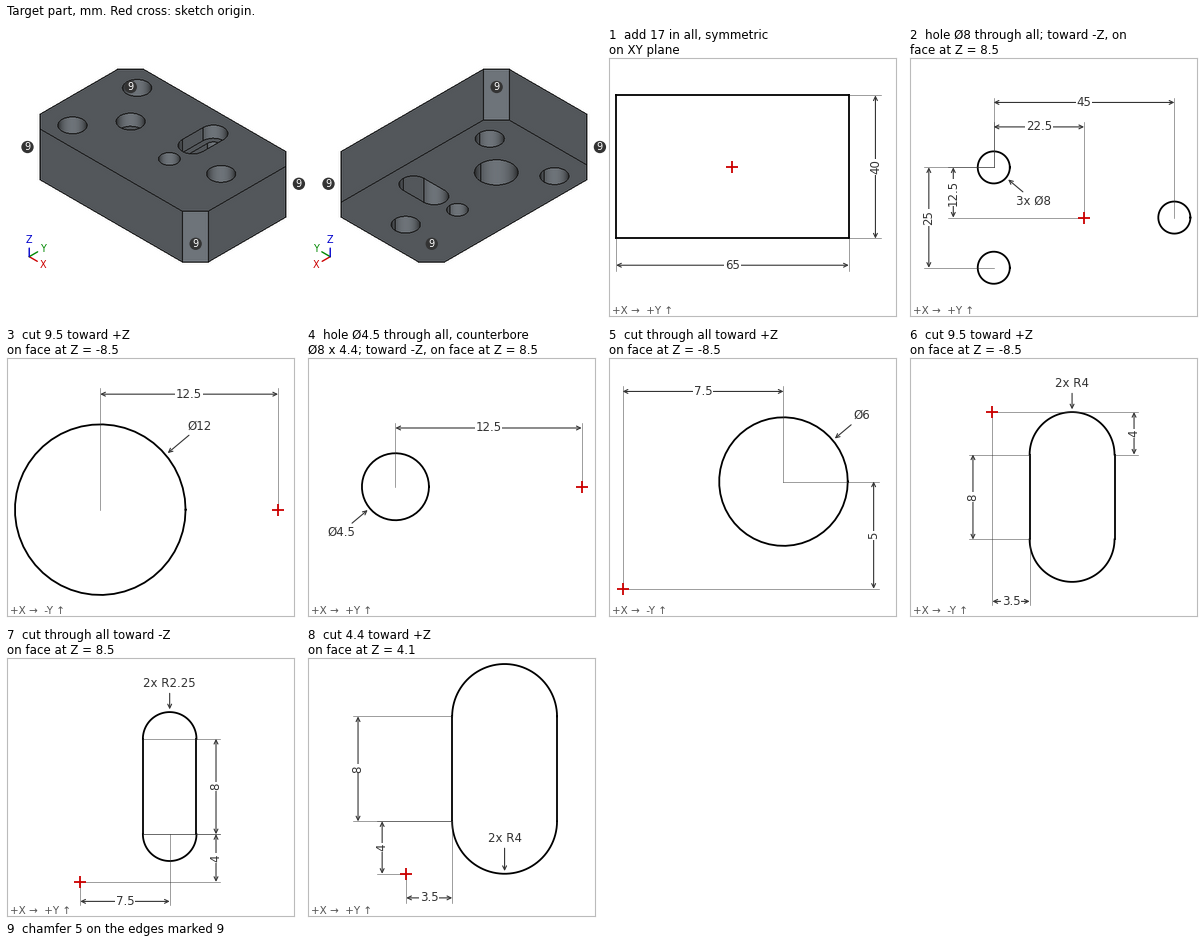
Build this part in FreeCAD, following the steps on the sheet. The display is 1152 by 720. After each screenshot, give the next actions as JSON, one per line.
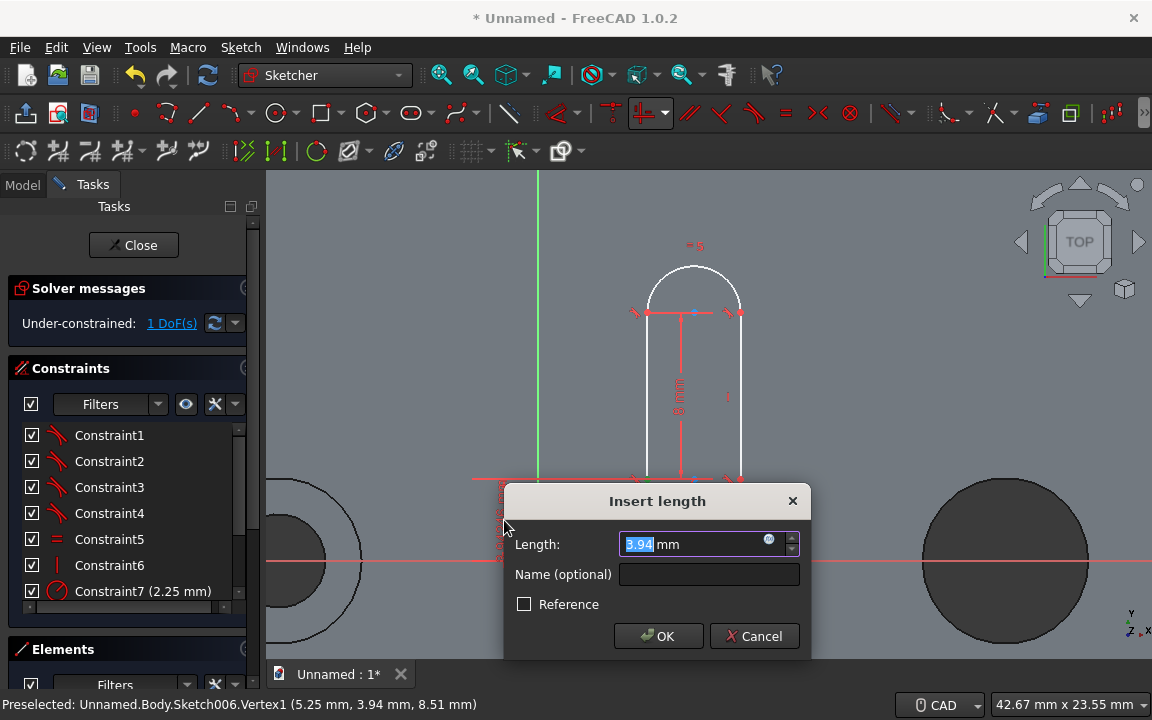
{"action": "type", "text": "4"}
{"action": "key", "text": "Return"}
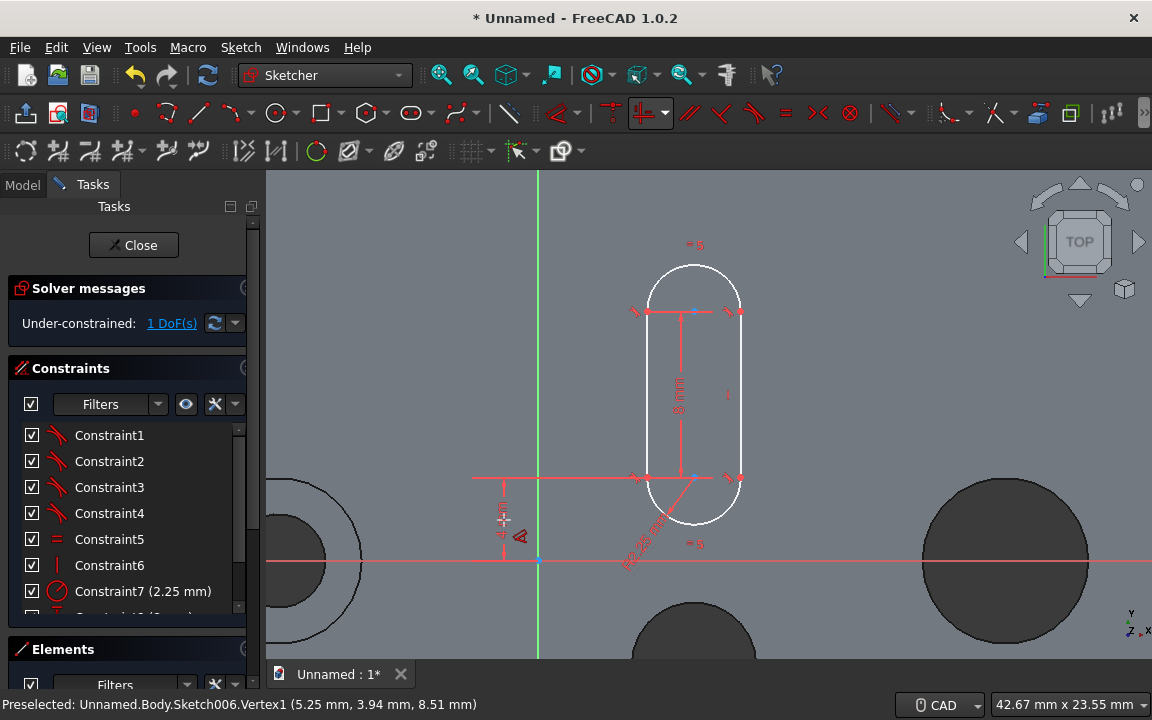
{"action": "left_click", "coordinate": [694, 478]}
{"action": "left_click", "coordinate": [616, 595]}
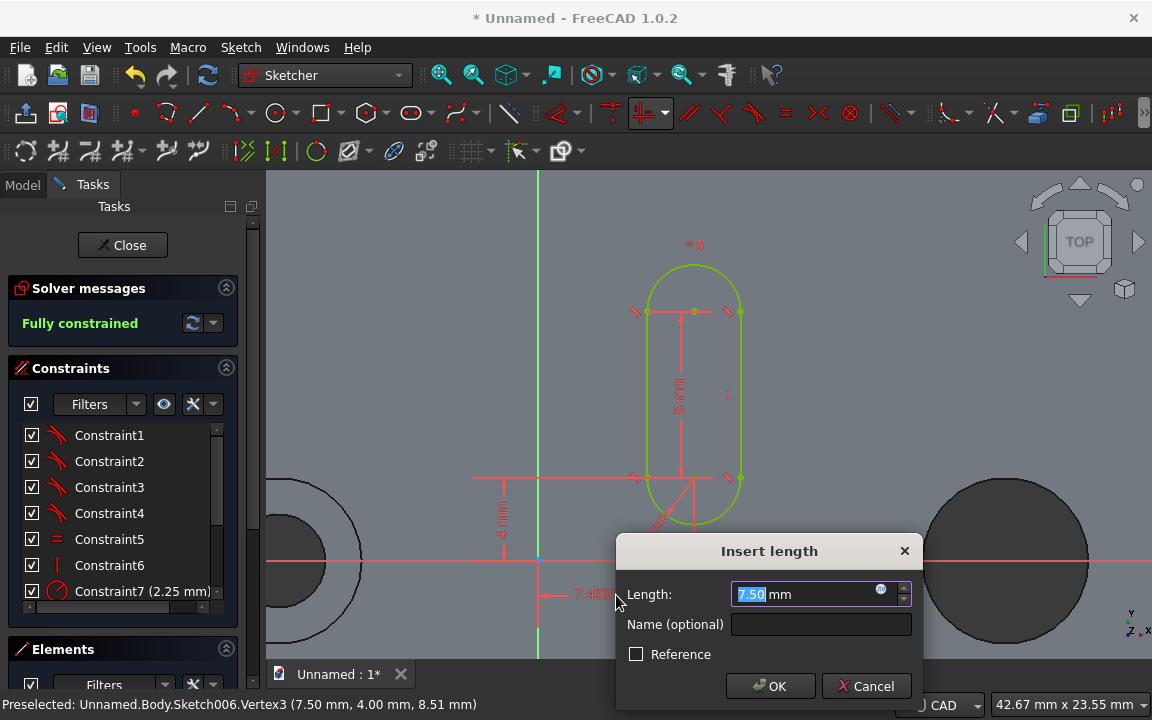
{"action": "type", "text": "7.5"}
{"action": "key", "text": "Return"}
{"action": "key", "text": "Escape"}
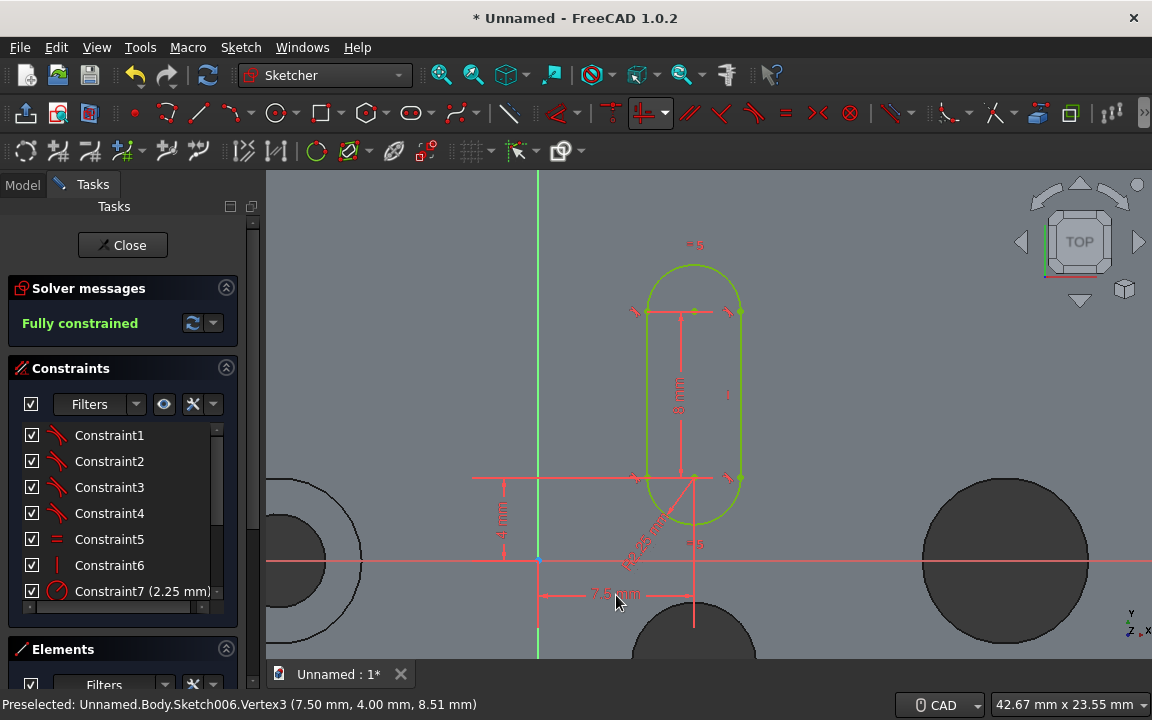
{"action": "left_click", "coordinate": [123, 245]}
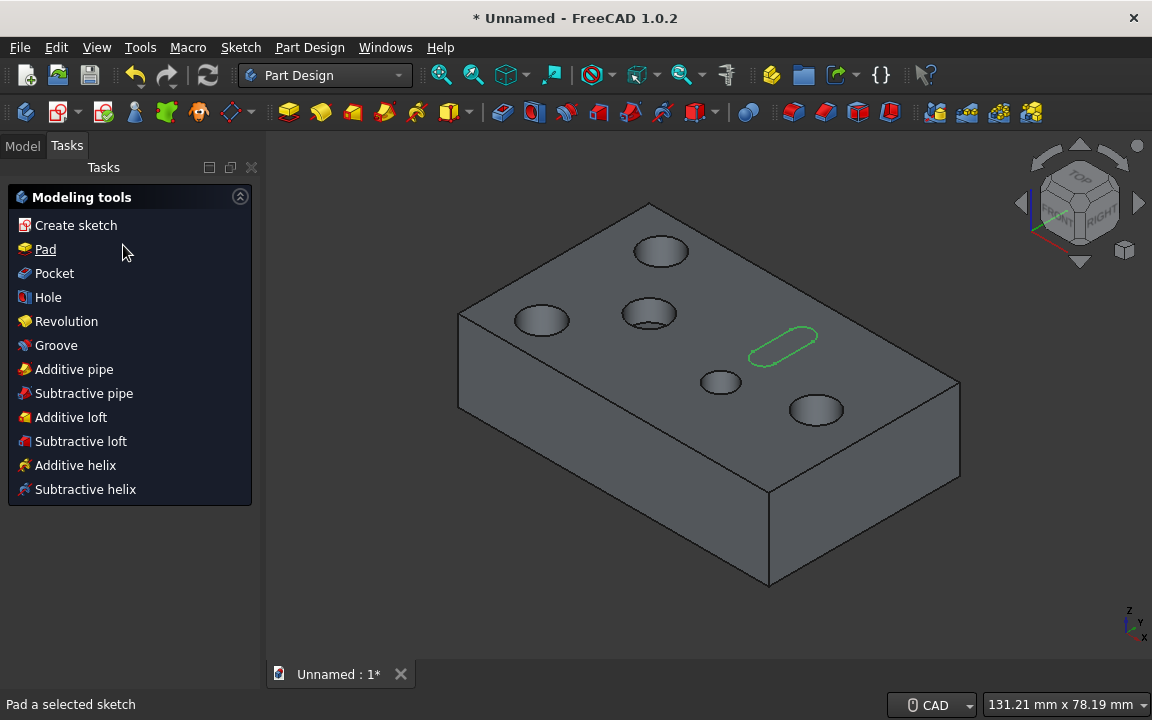
{"action": "left_click", "coordinate": [504, 112]}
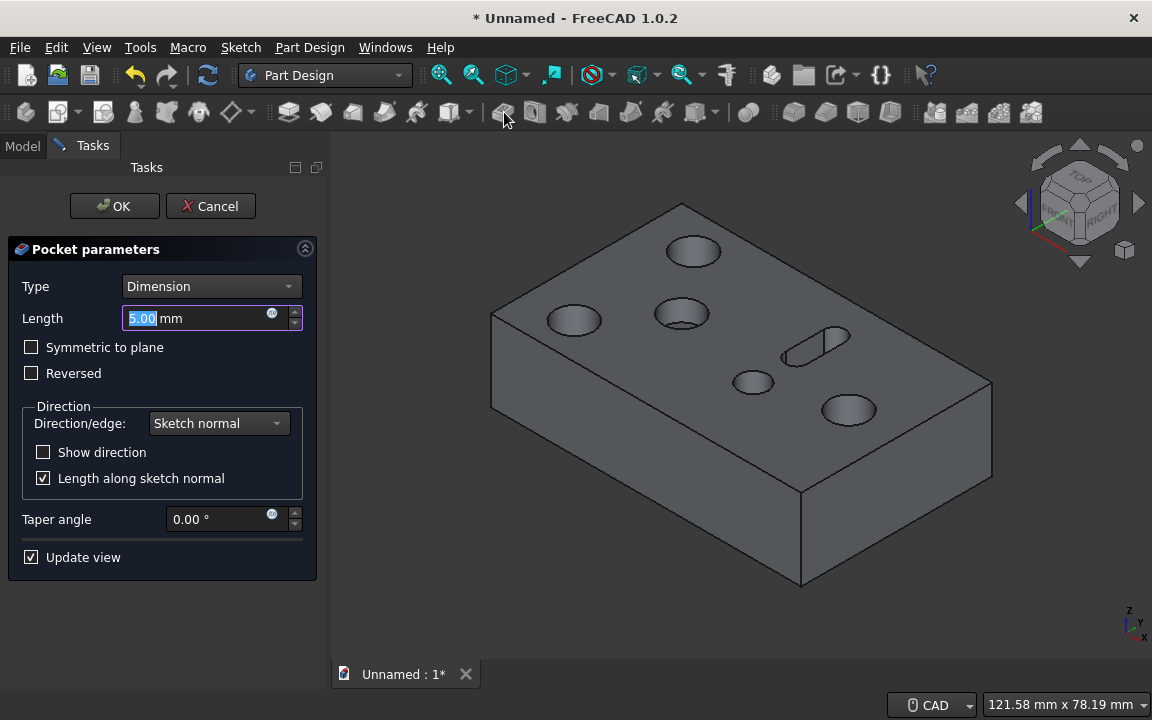
{"action": "left_click", "coordinate": [212, 286]}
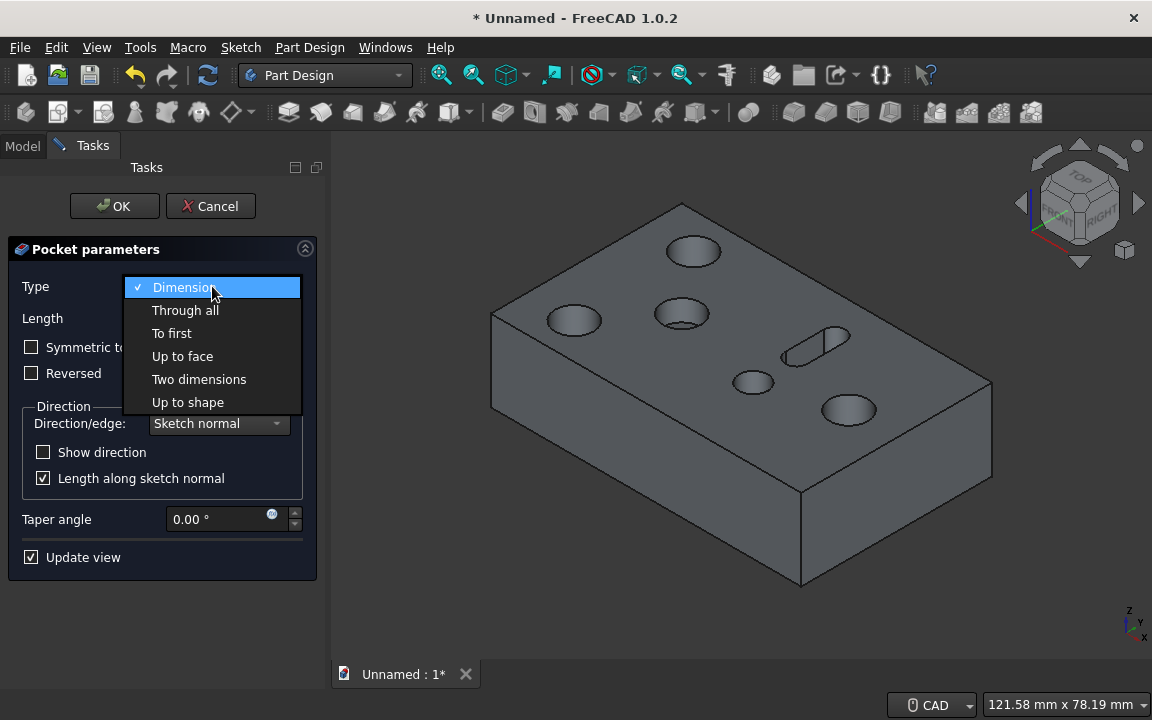
{"action": "left_click", "coordinate": [212, 310]}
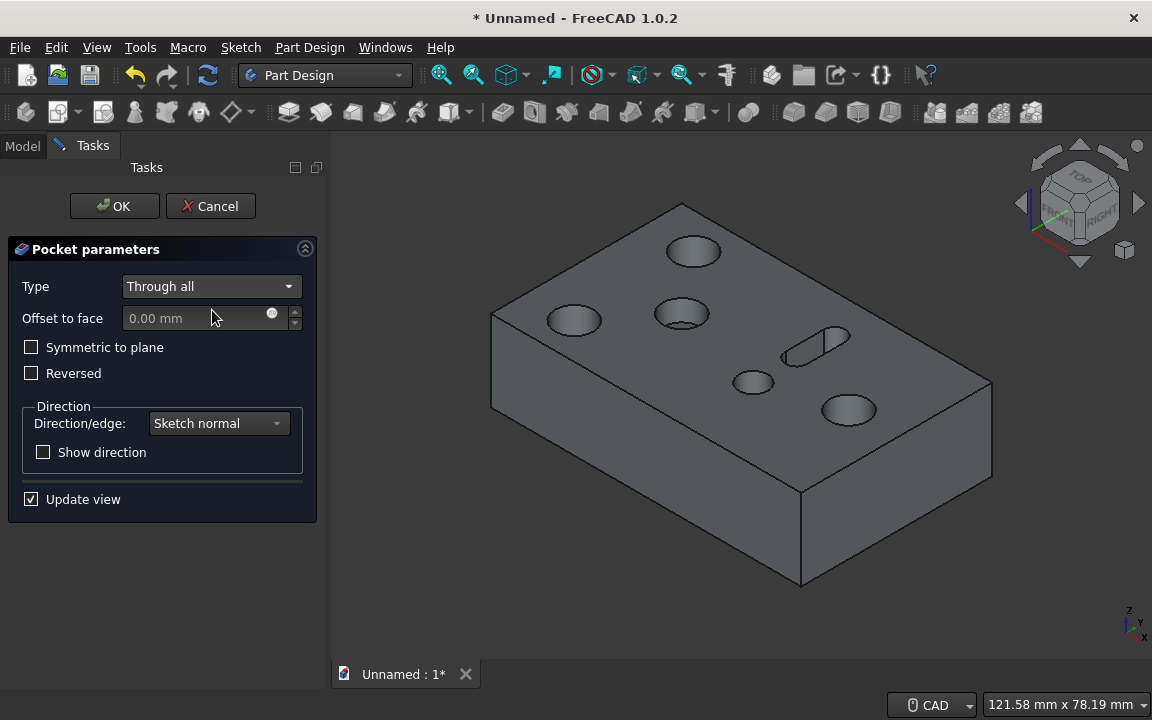
{"action": "left_click", "coordinate": [115, 206]}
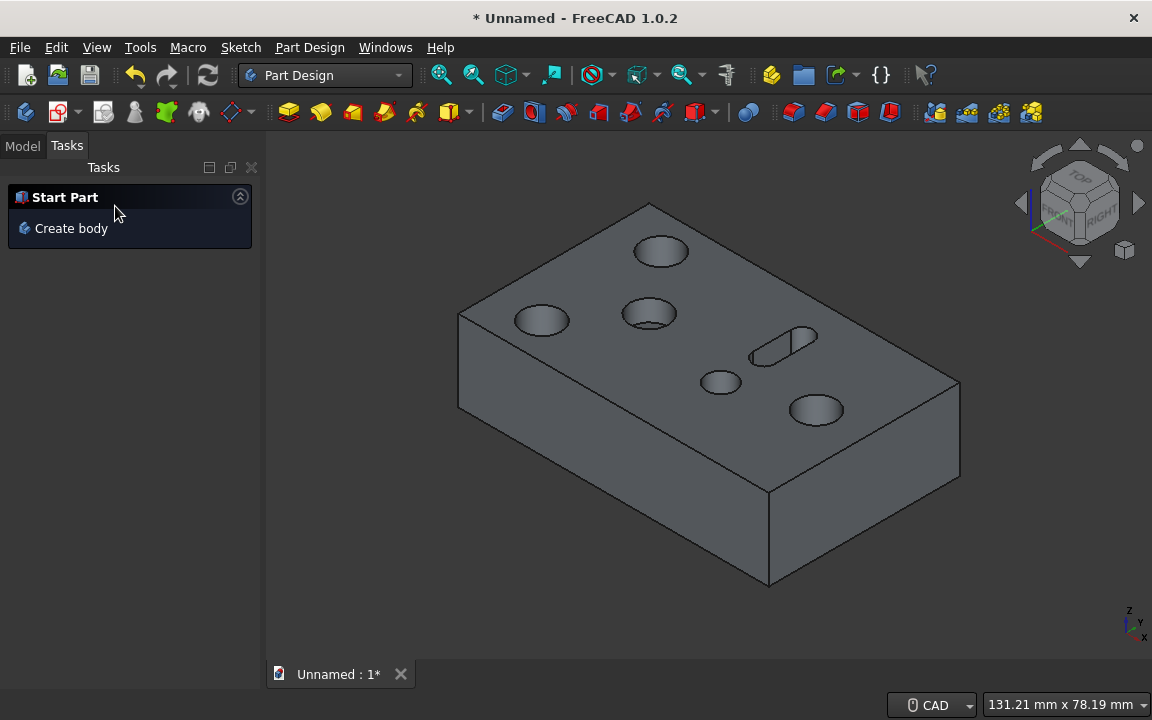
{"action": "scroll", "coordinate": [627, 337], "scroll_direction": "up", "scroll_amount": 5}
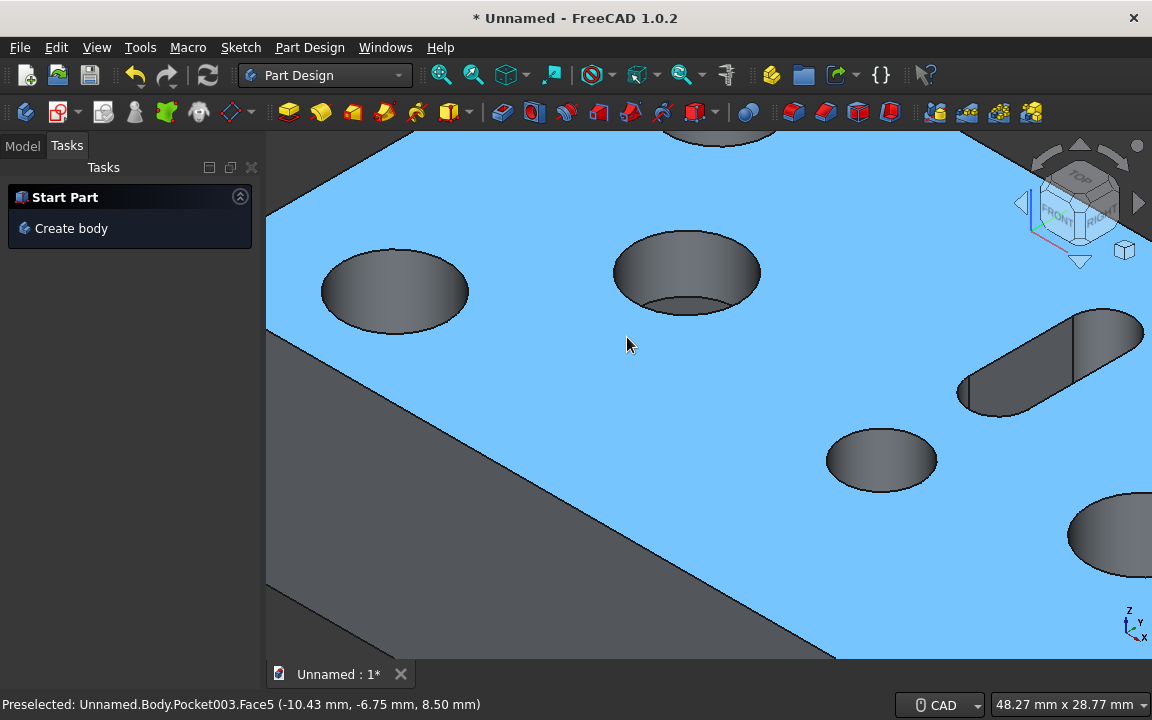
{"action": "left_click", "coordinate": [687, 304]}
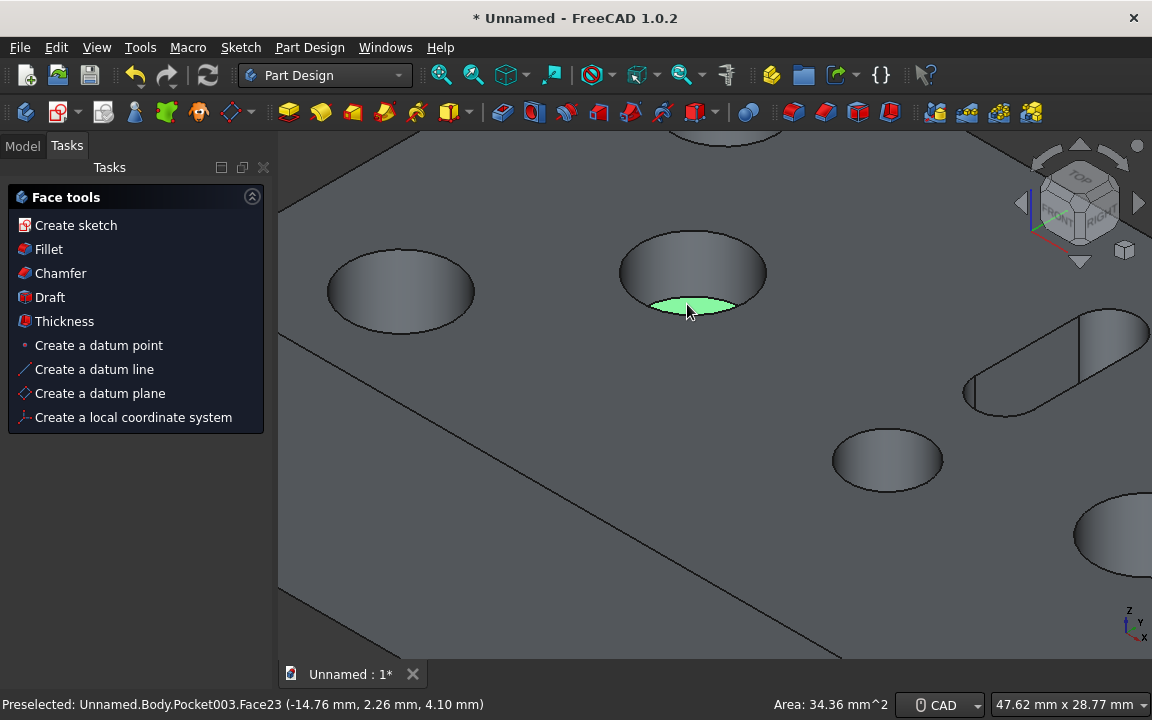
{"action": "left_click", "coordinate": [58, 112]}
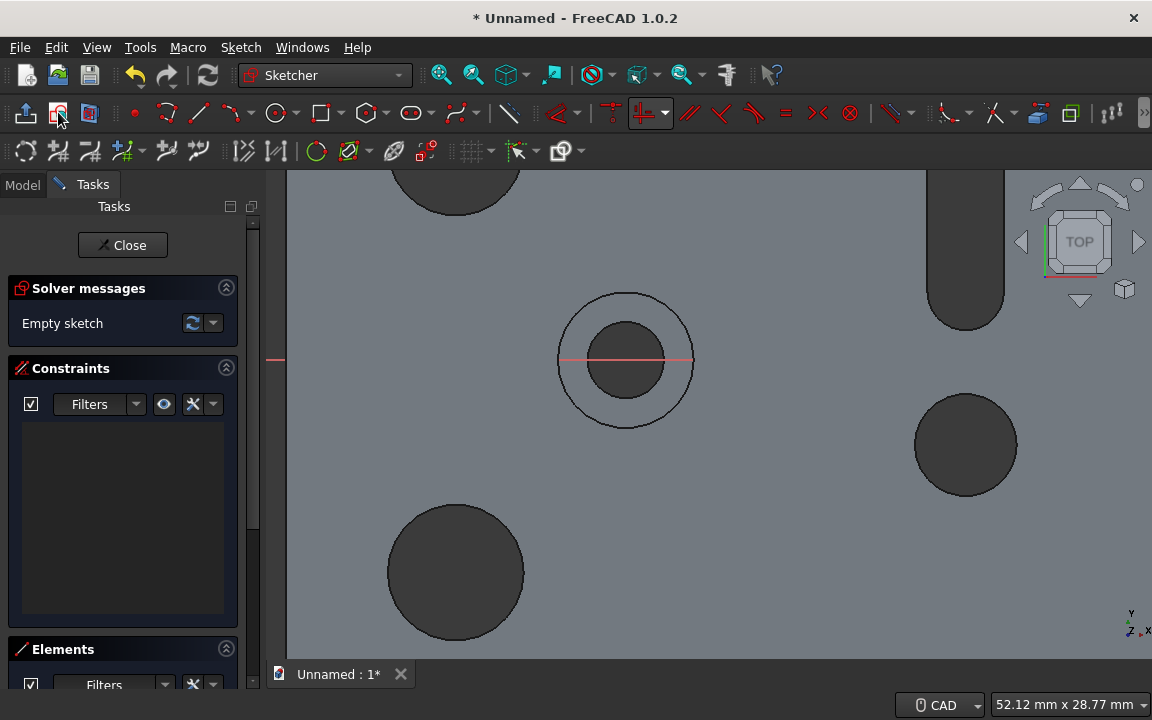
{"action": "scroll", "coordinate": [294, 631], "scroll_direction": "down", "scroll_amount": 2}